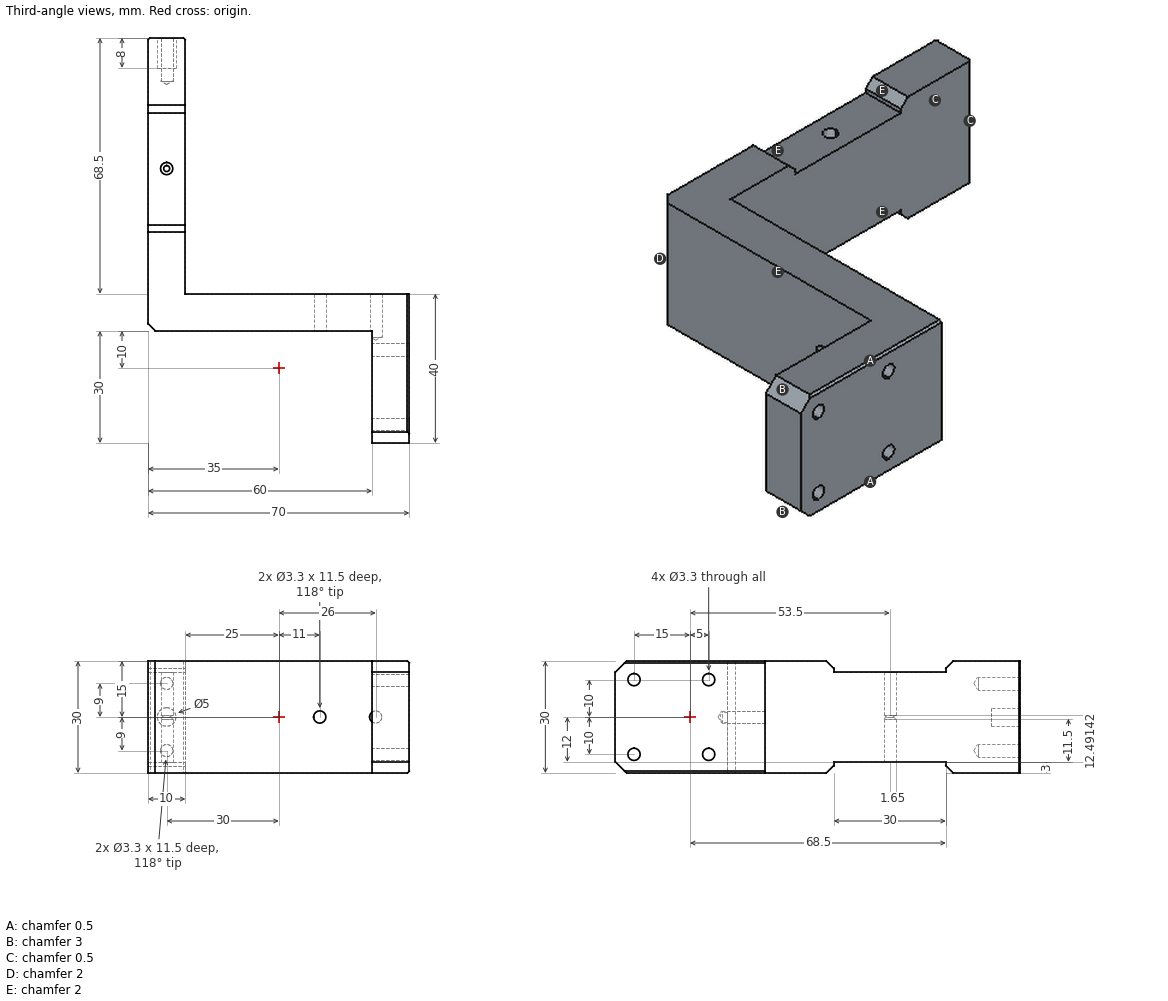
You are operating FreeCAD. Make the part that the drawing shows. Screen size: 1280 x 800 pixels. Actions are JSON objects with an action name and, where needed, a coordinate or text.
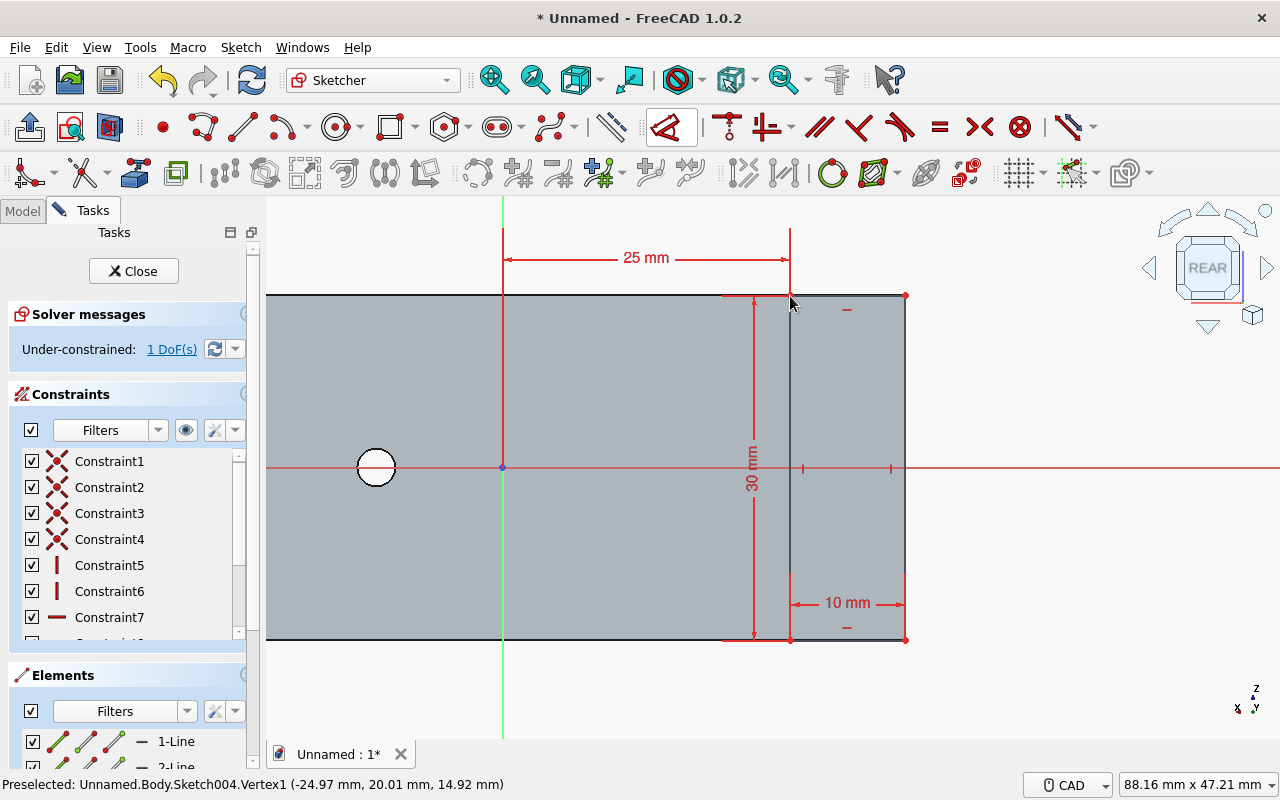
{"action": "left_click", "coordinate": [790, 296]}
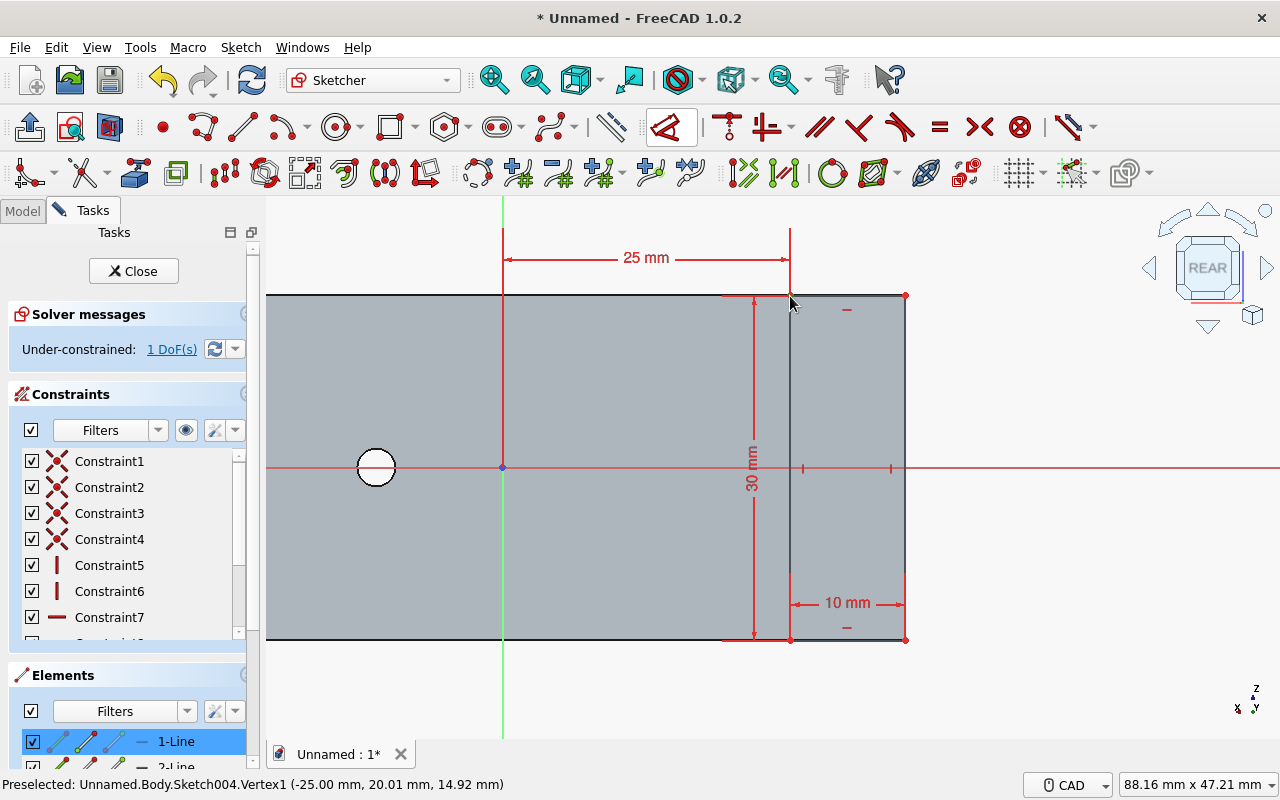
{"action": "key", "text": "i"}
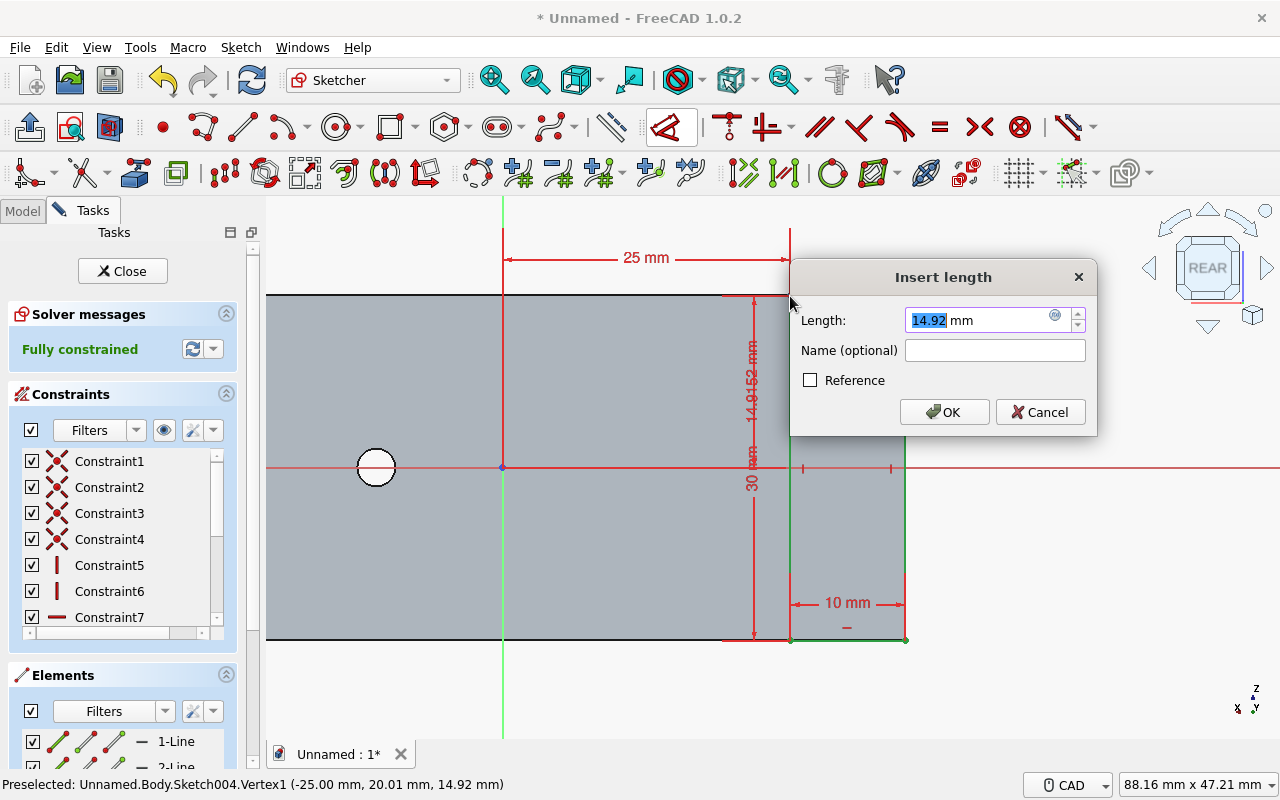
{"action": "type", "text": "15"}
{"action": "key", "text": "Return"}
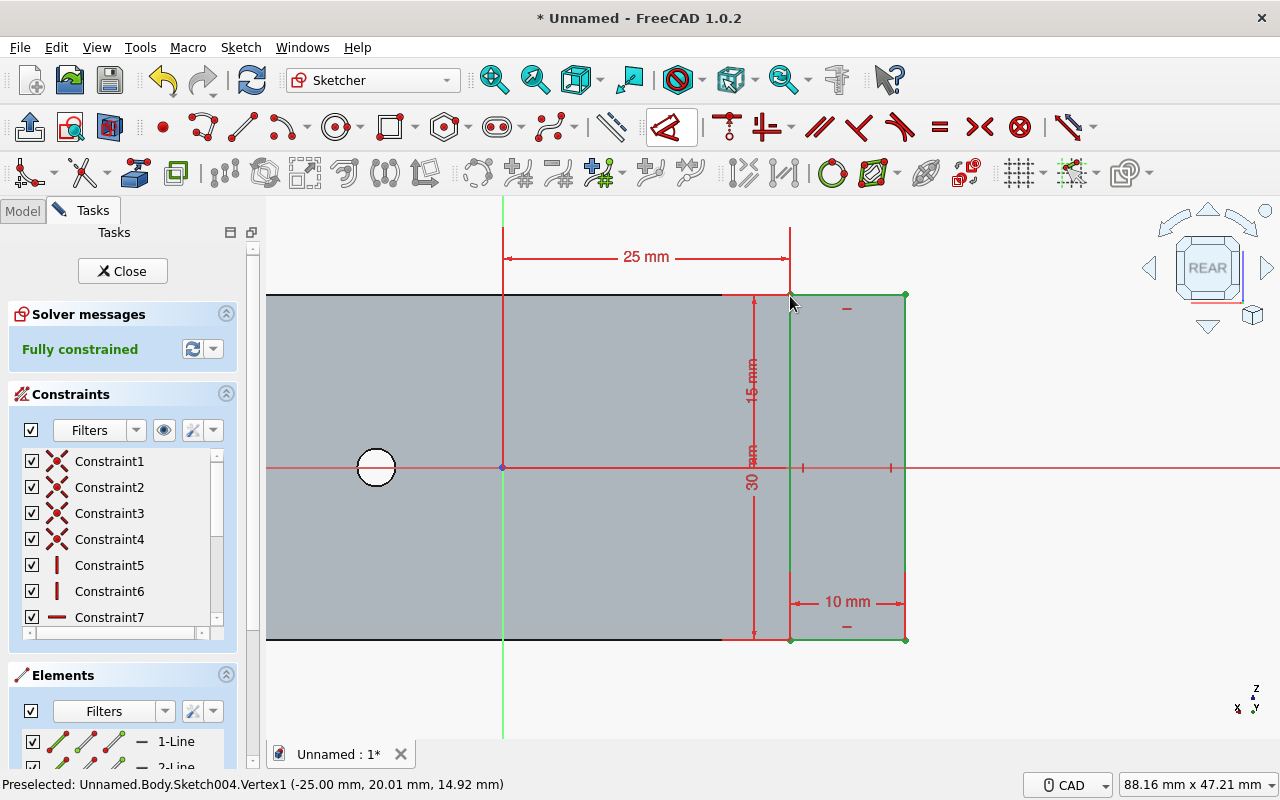
{"action": "left_click", "coordinate": [123, 271]}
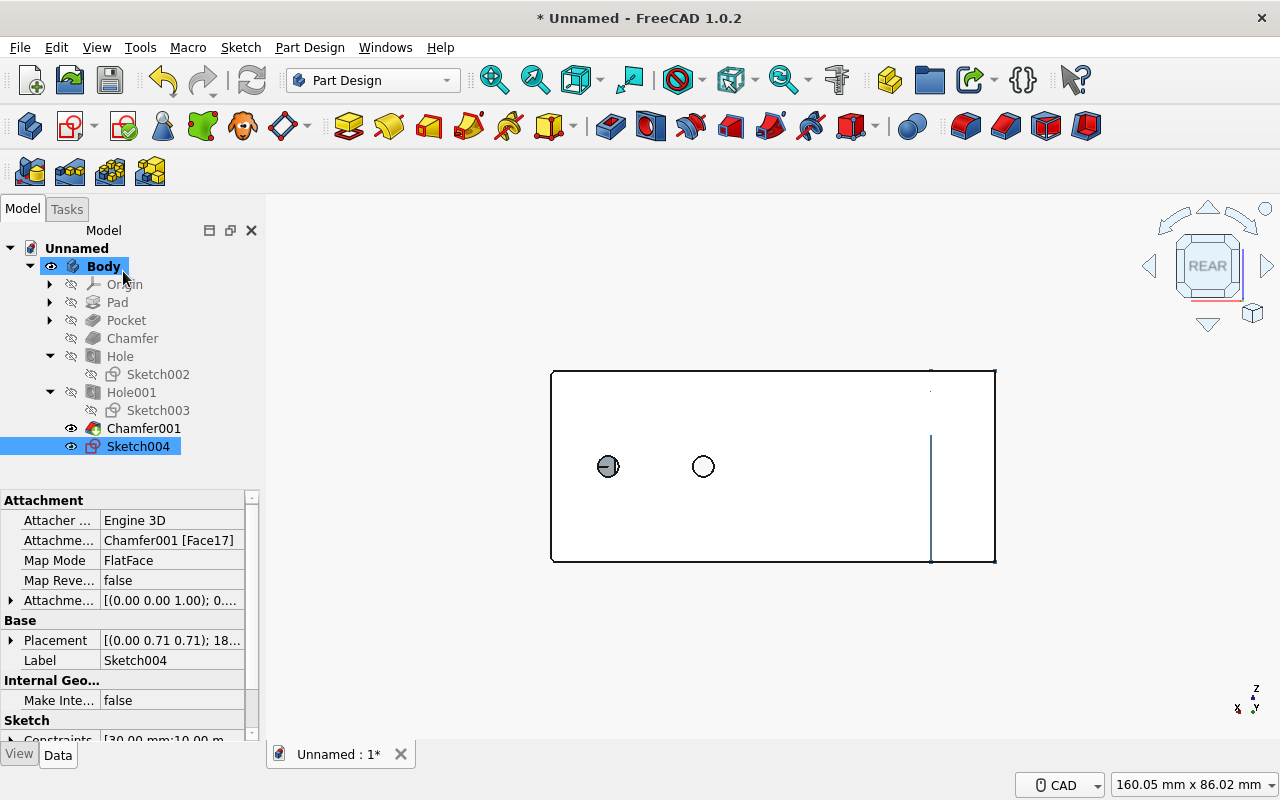
{"action": "left_click", "coordinate": [350, 126]}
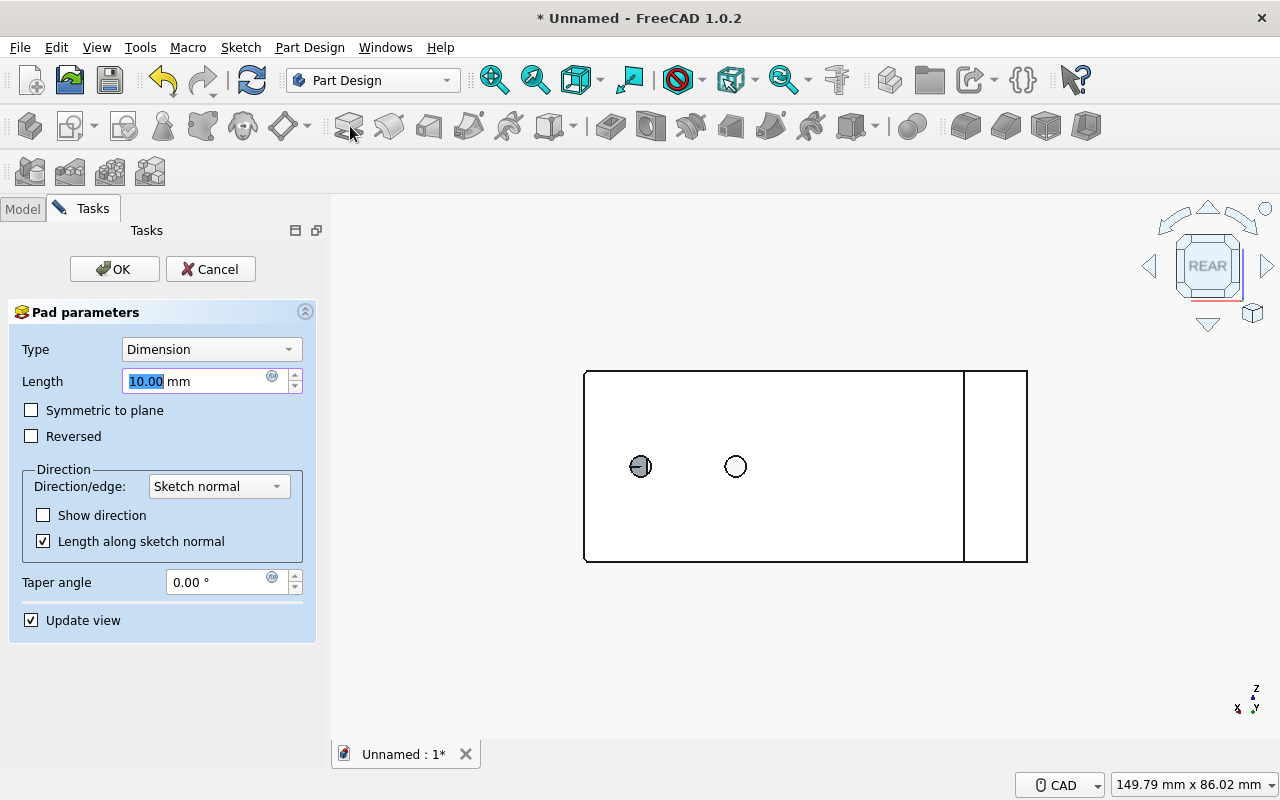
{"action": "type", "text": "68.5"}
{"action": "key", "text": "Tab"}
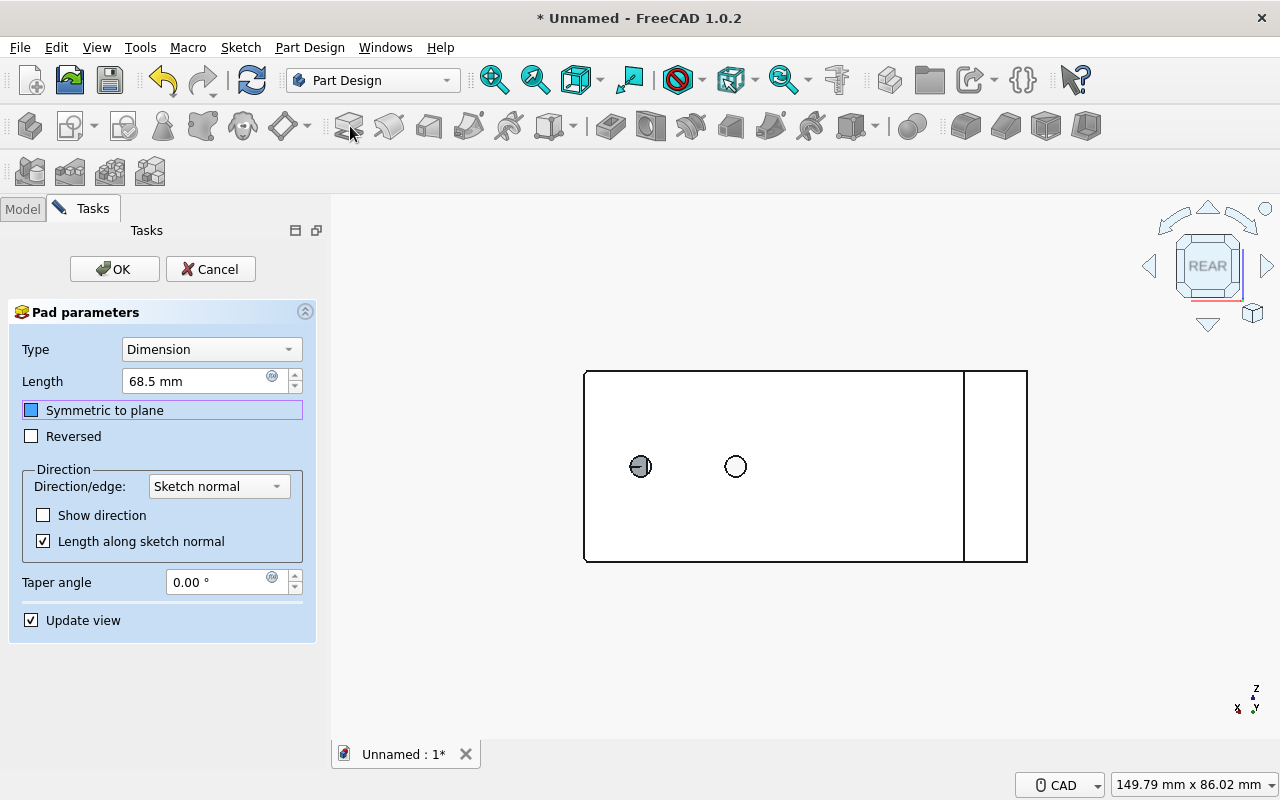
{"action": "left_click", "coordinate": [115, 269]}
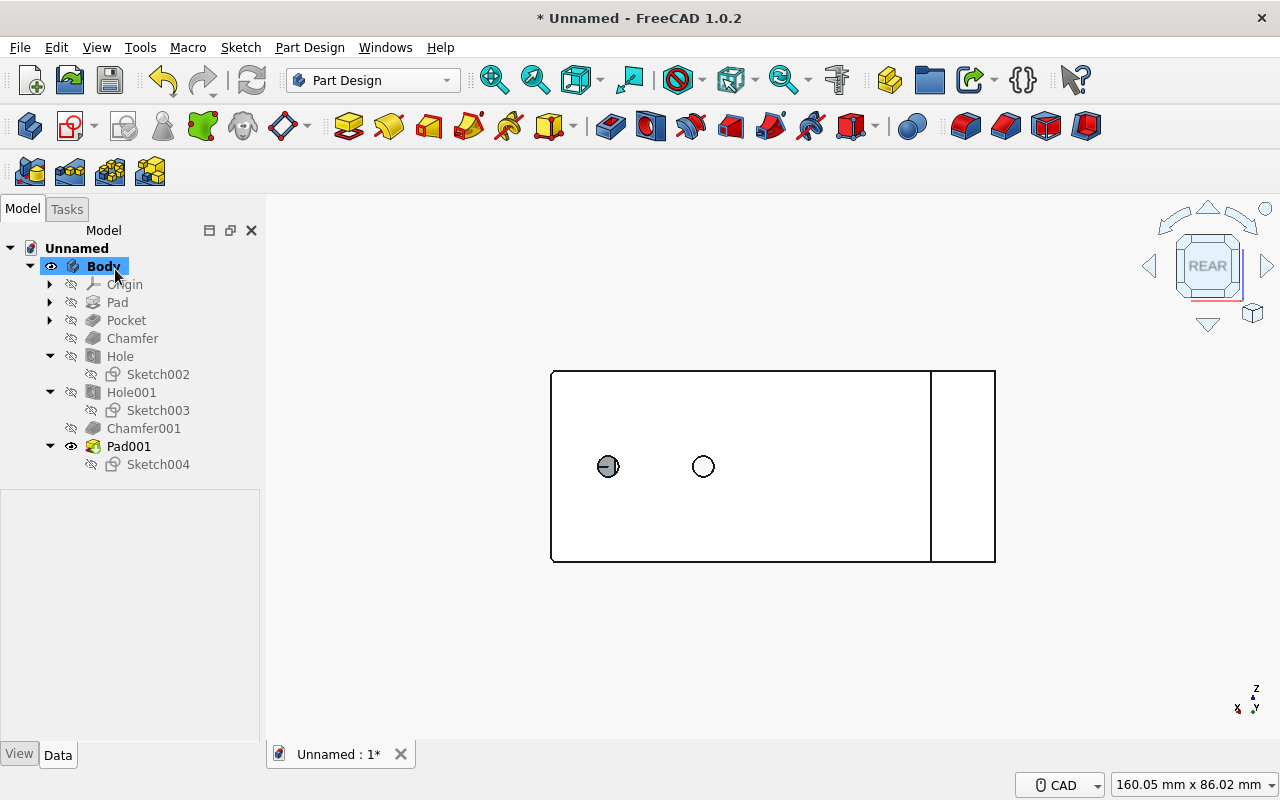
{"action": "left_click", "coordinate": [496, 80]}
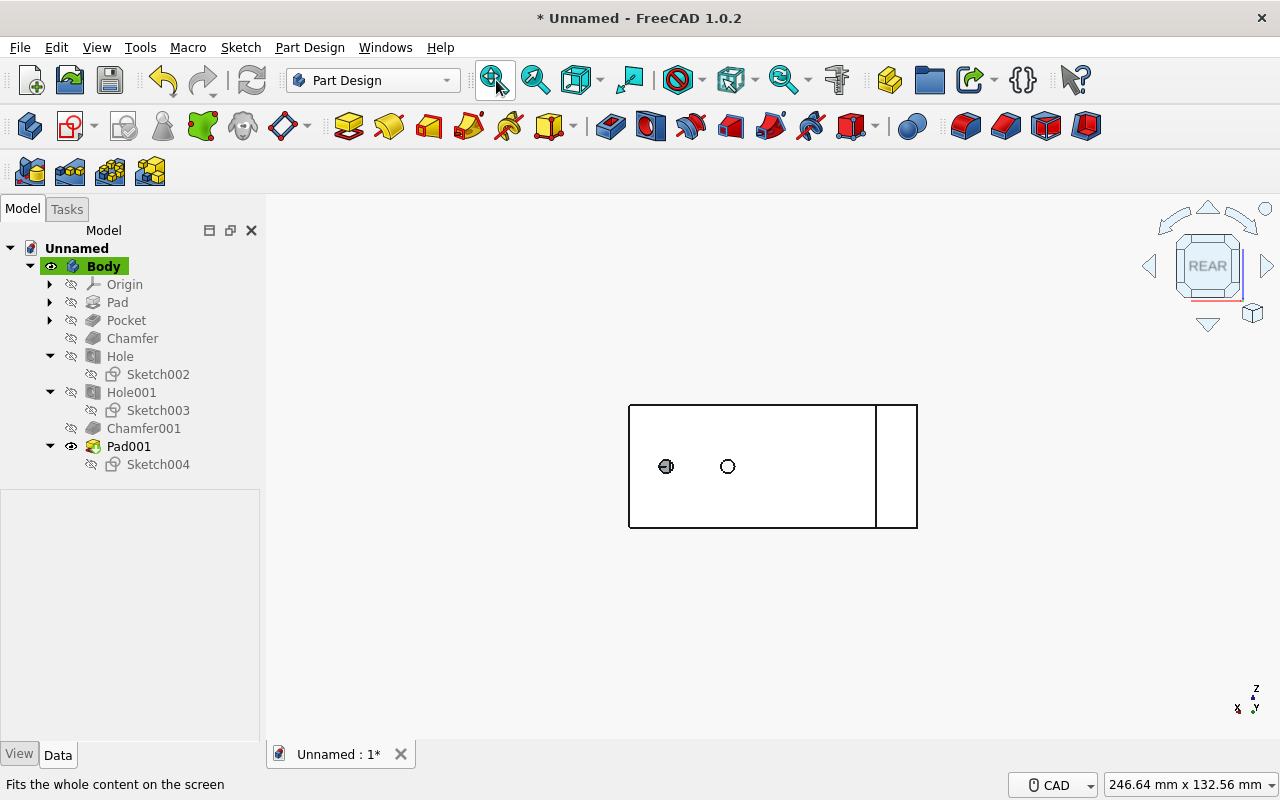
{"action": "left_click", "coordinate": [917, 465]}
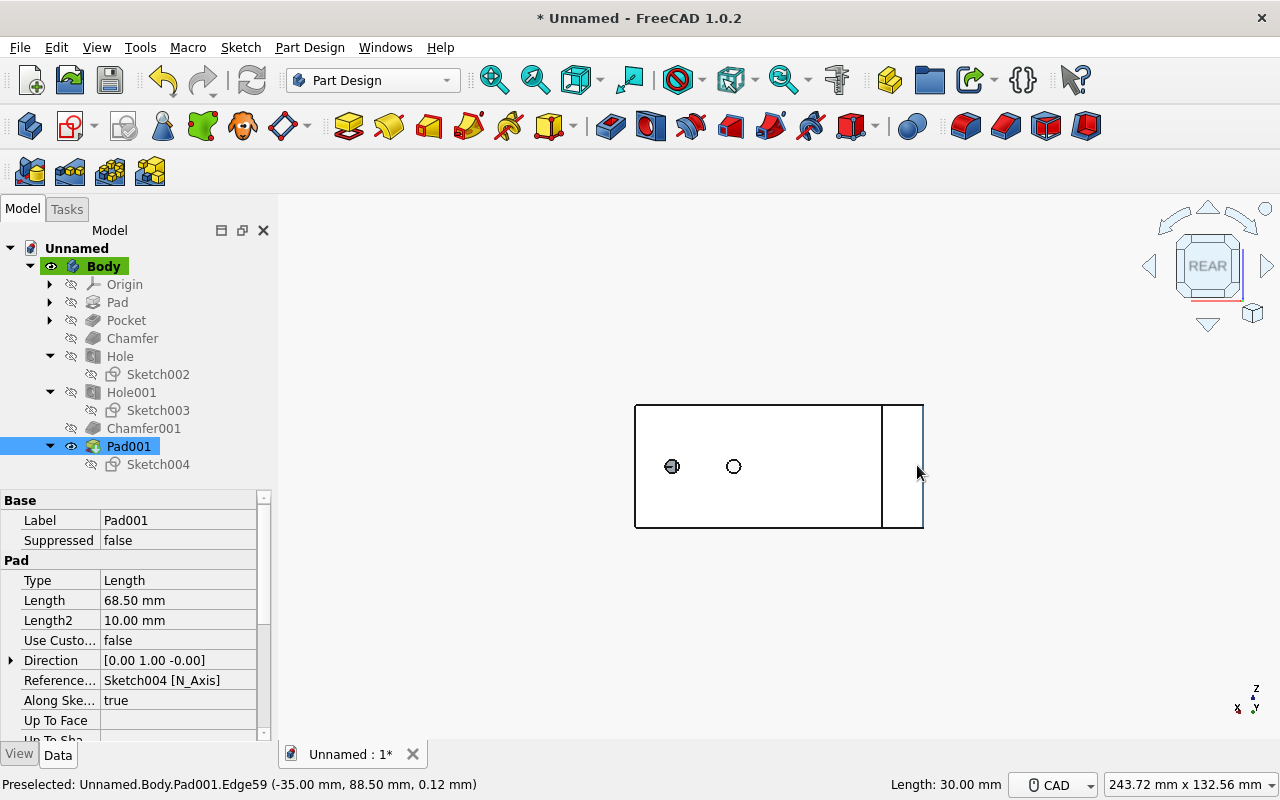
{"action": "key", "text": "0"}